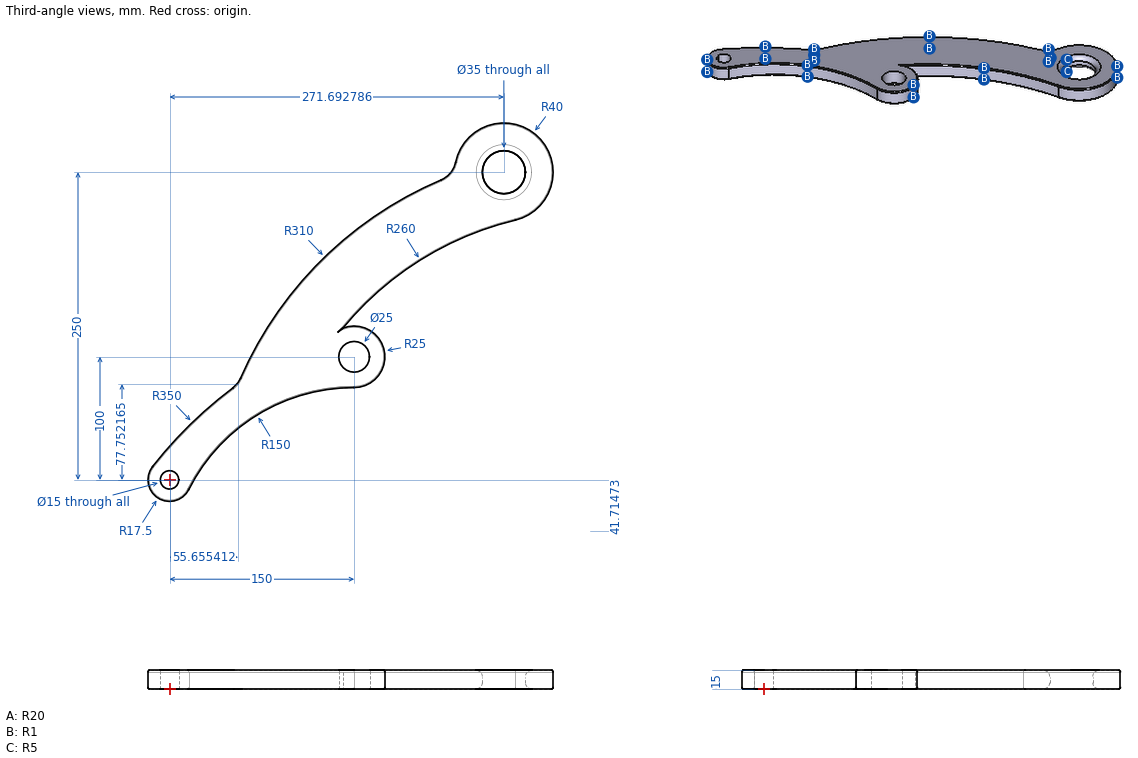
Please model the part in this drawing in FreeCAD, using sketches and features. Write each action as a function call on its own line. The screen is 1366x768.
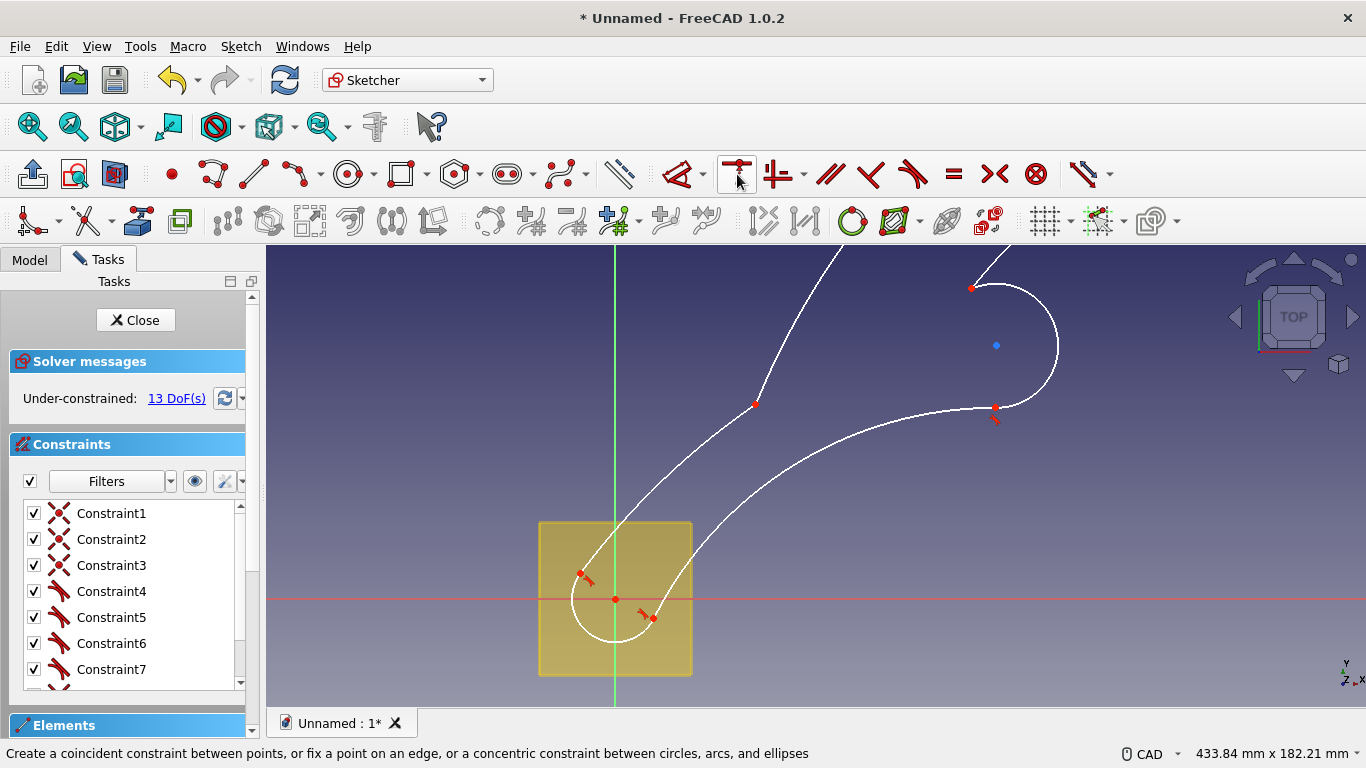
click(676, 174)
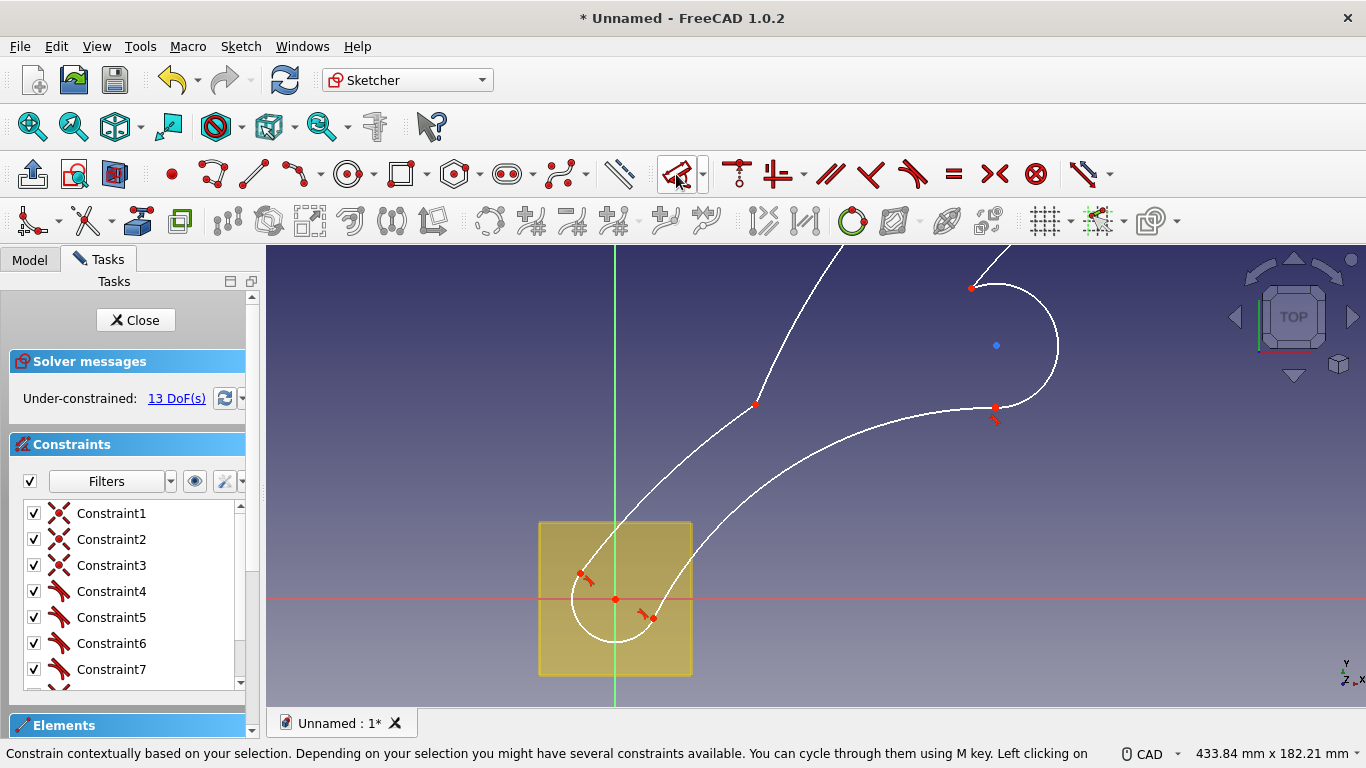
click(575, 614)
click(545, 625)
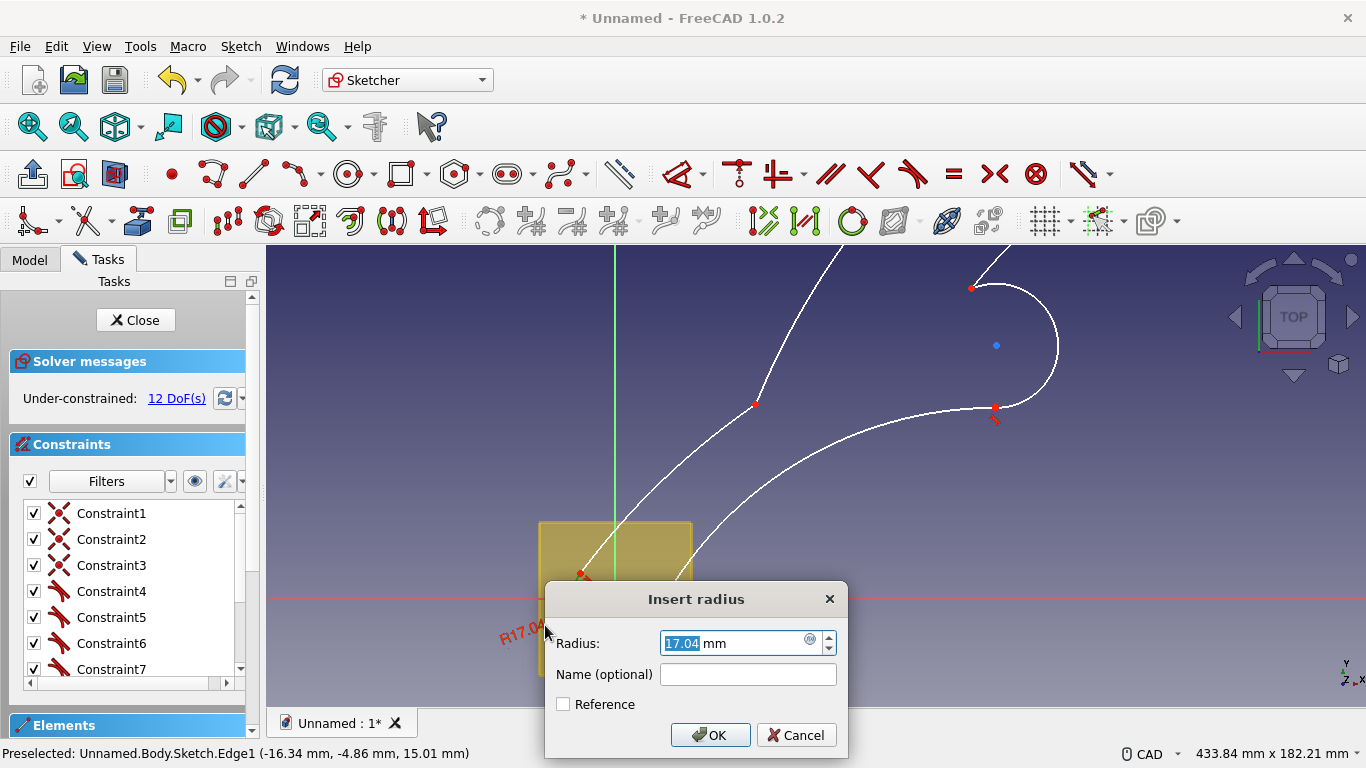
text(17.5)
key(Return)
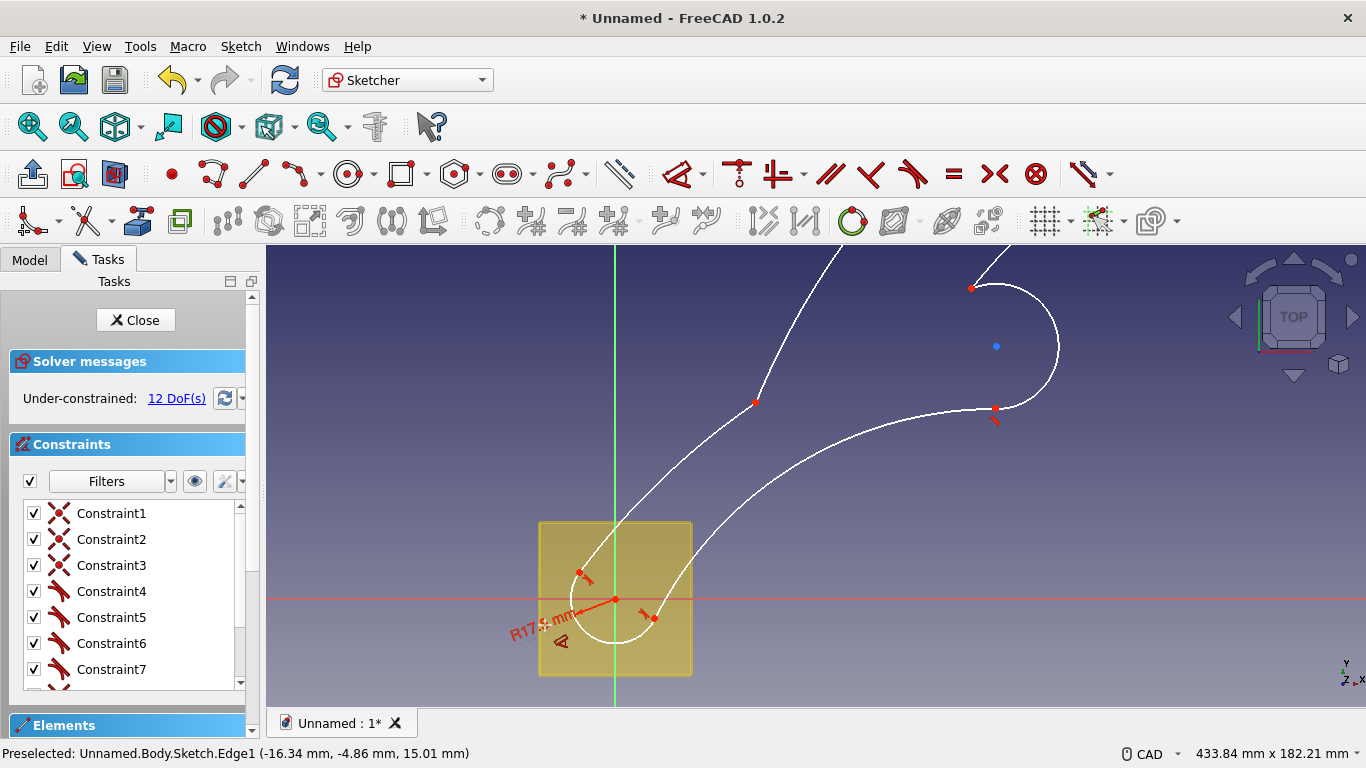
click(872, 430)
click(862, 400)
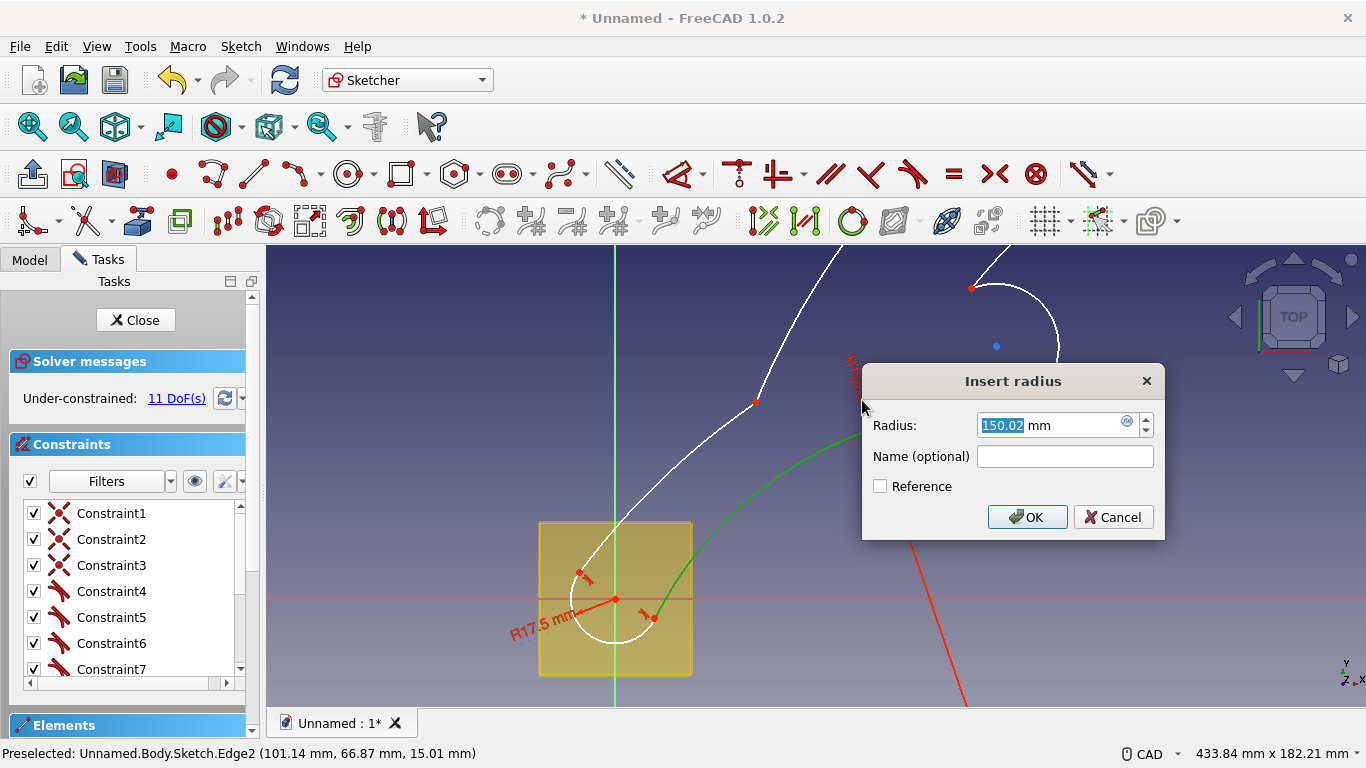
text(150)
key(Return)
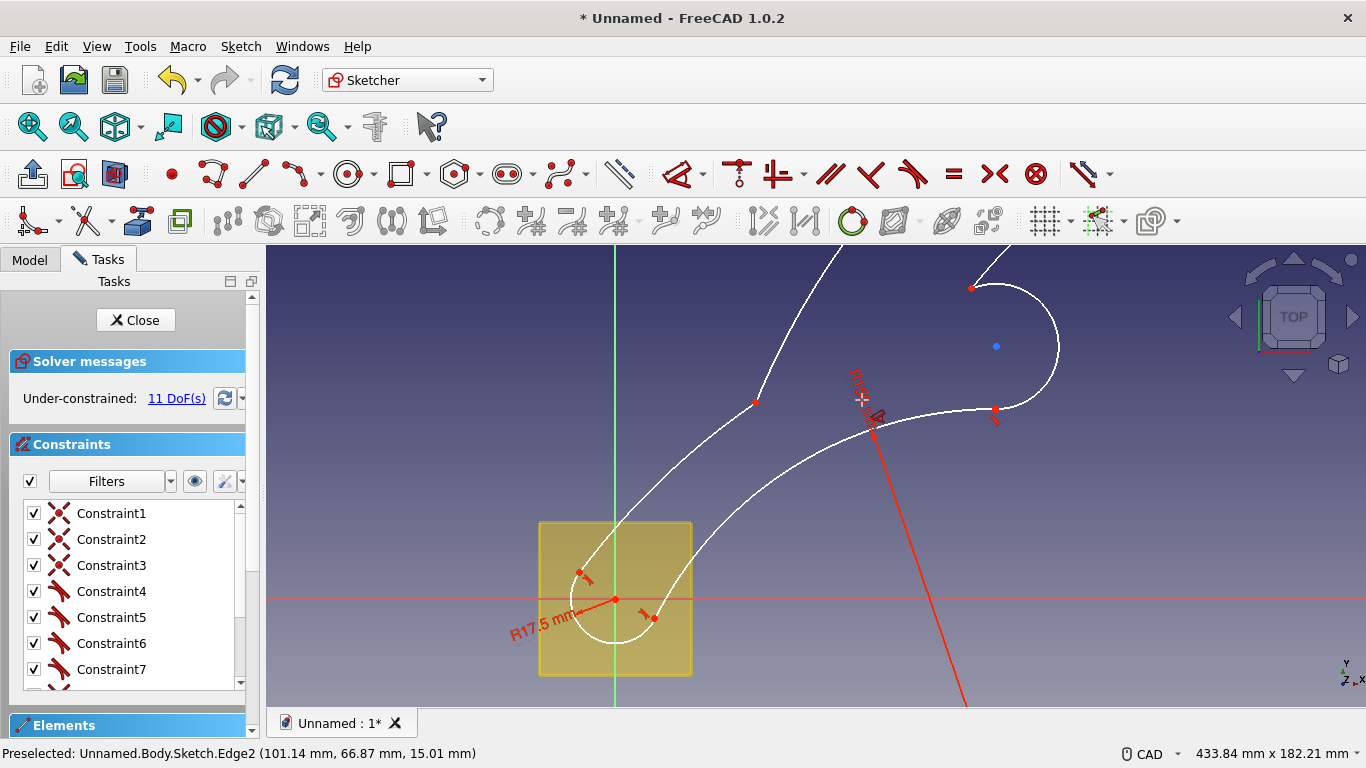
click(1051, 377)
click(1079, 393)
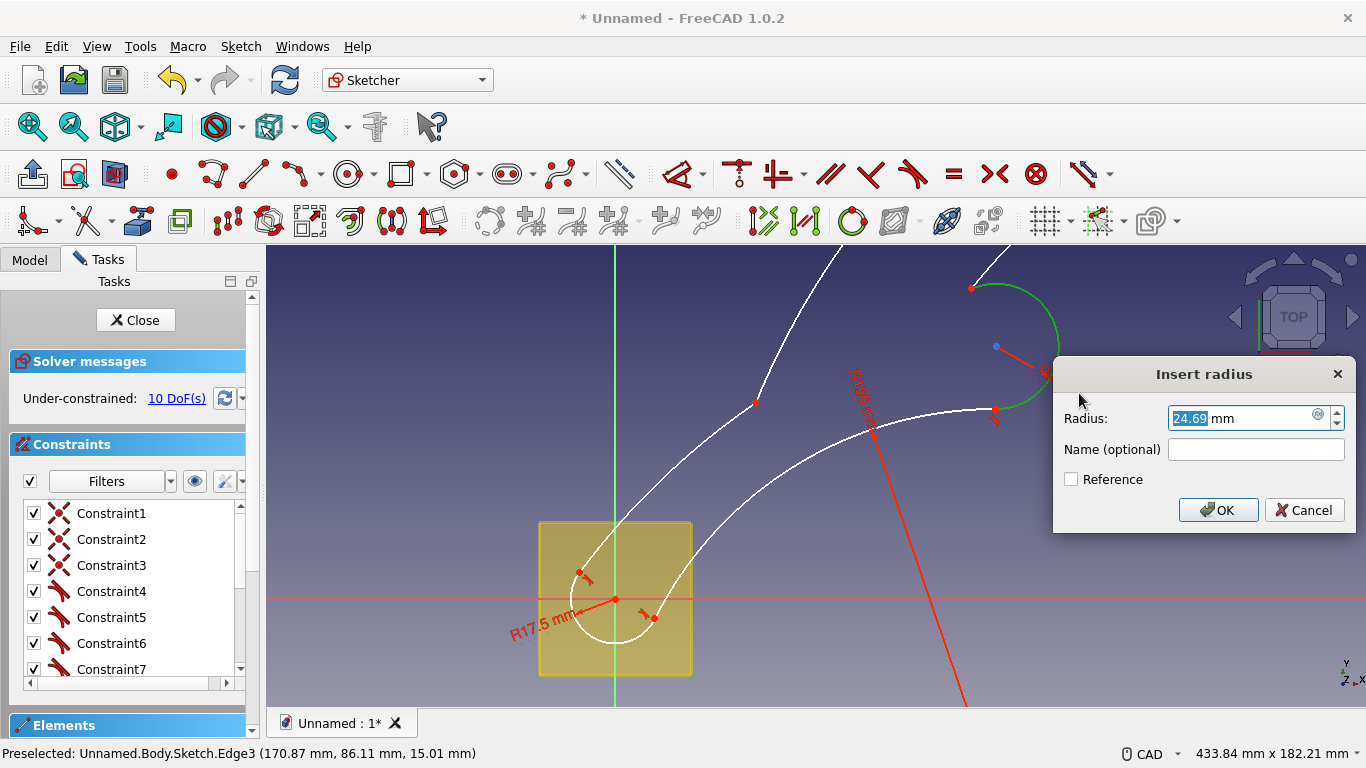
text(25)
key(Return)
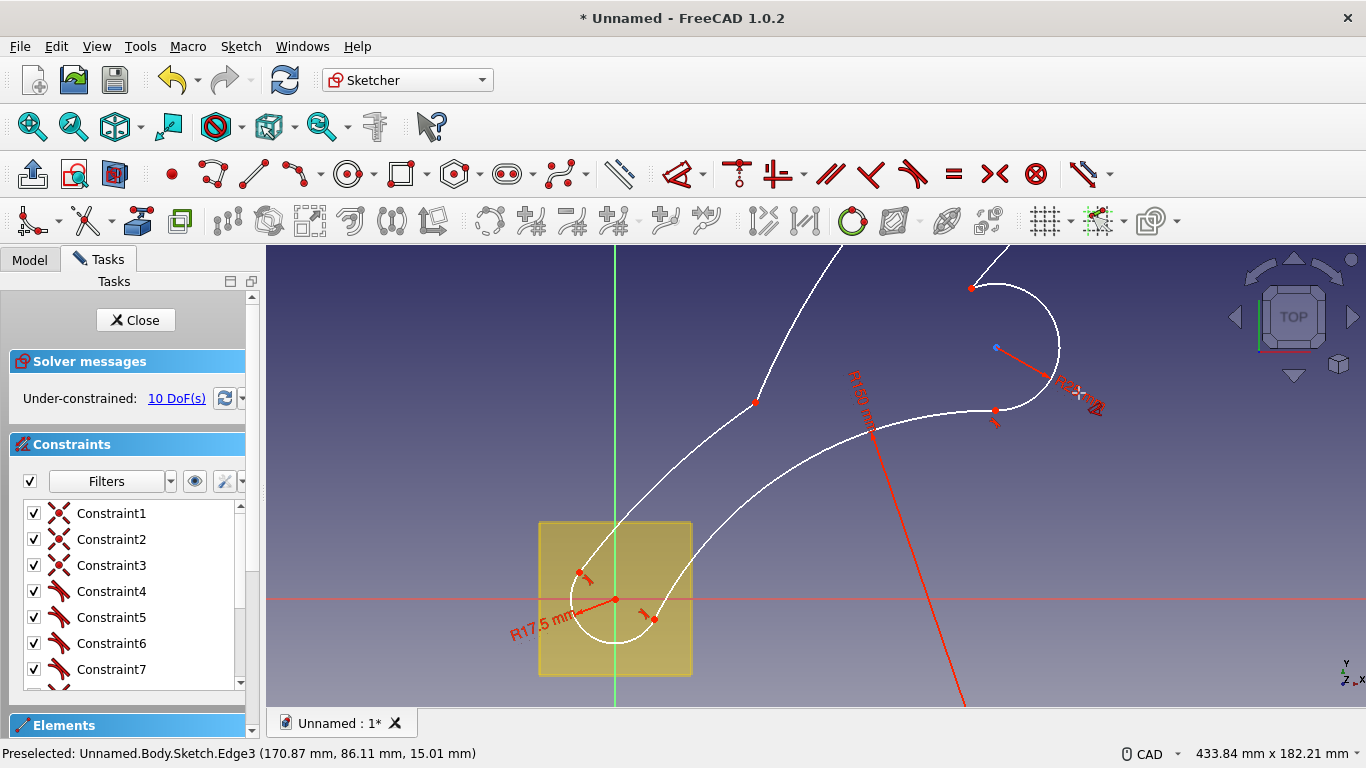
scroll(616, 602, down, 5)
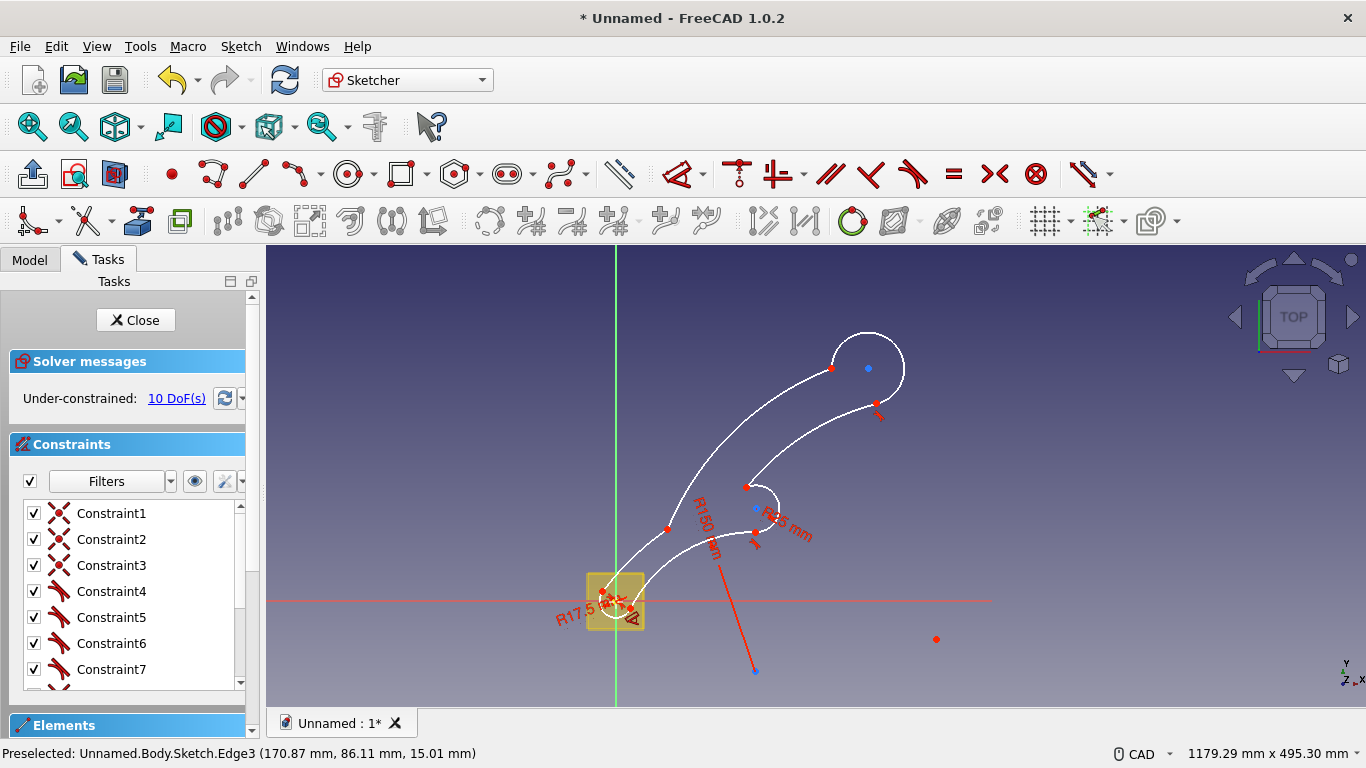
click(833, 420)
click(819, 391)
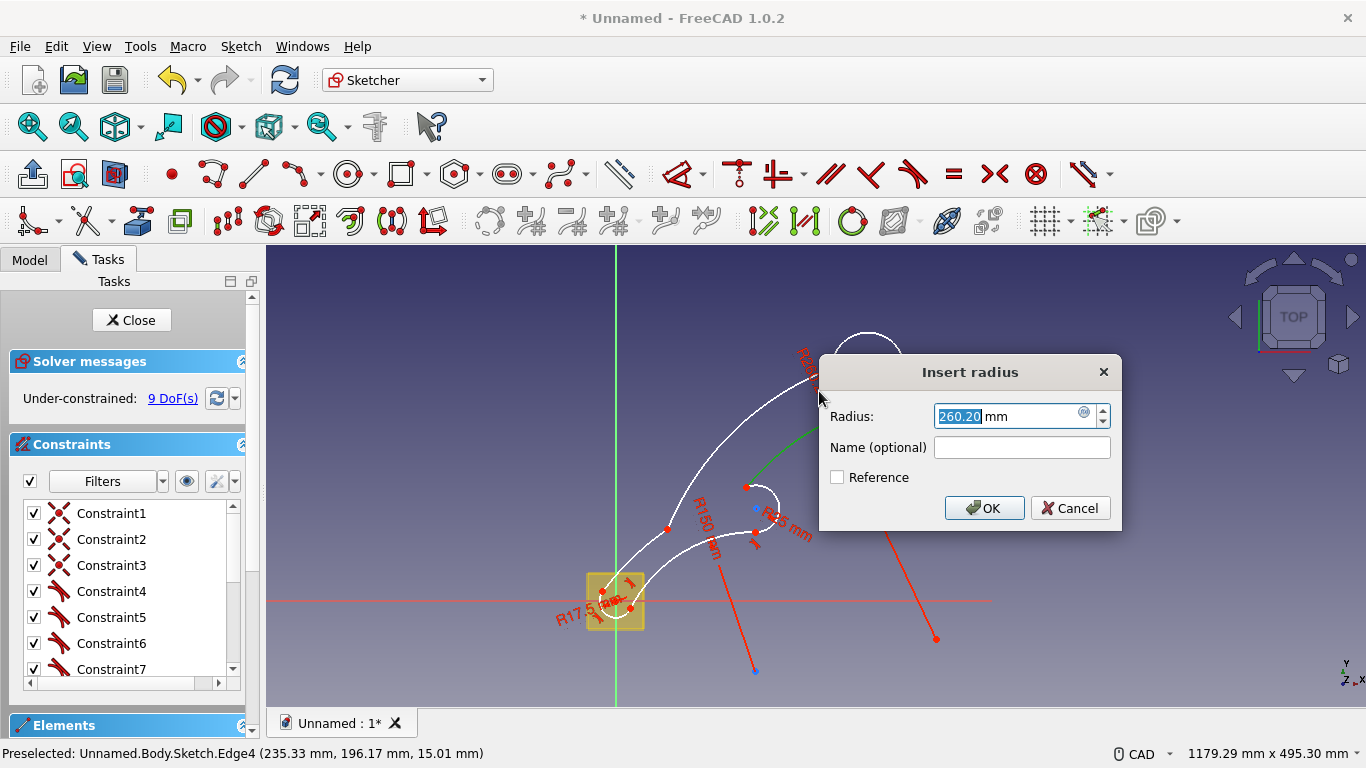
text(260)
key(Return)